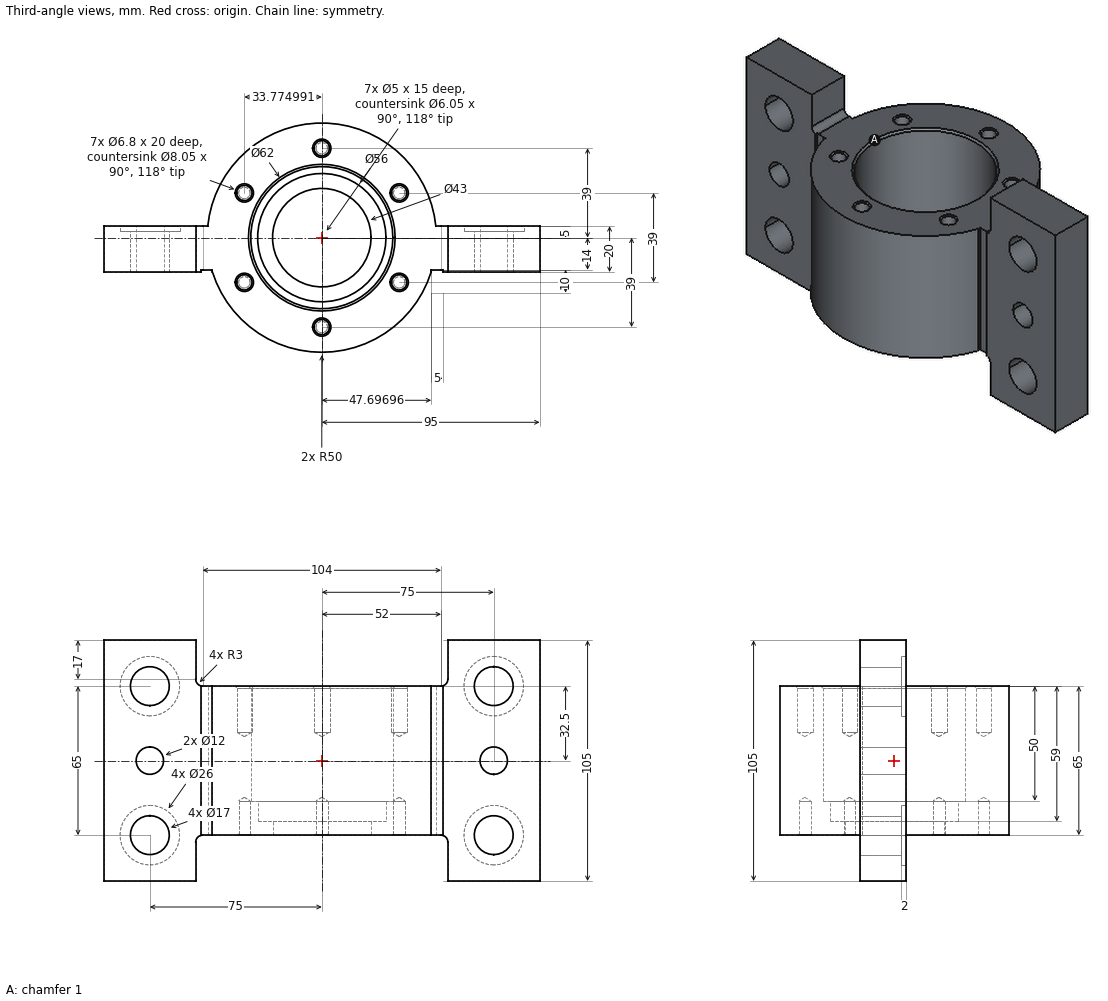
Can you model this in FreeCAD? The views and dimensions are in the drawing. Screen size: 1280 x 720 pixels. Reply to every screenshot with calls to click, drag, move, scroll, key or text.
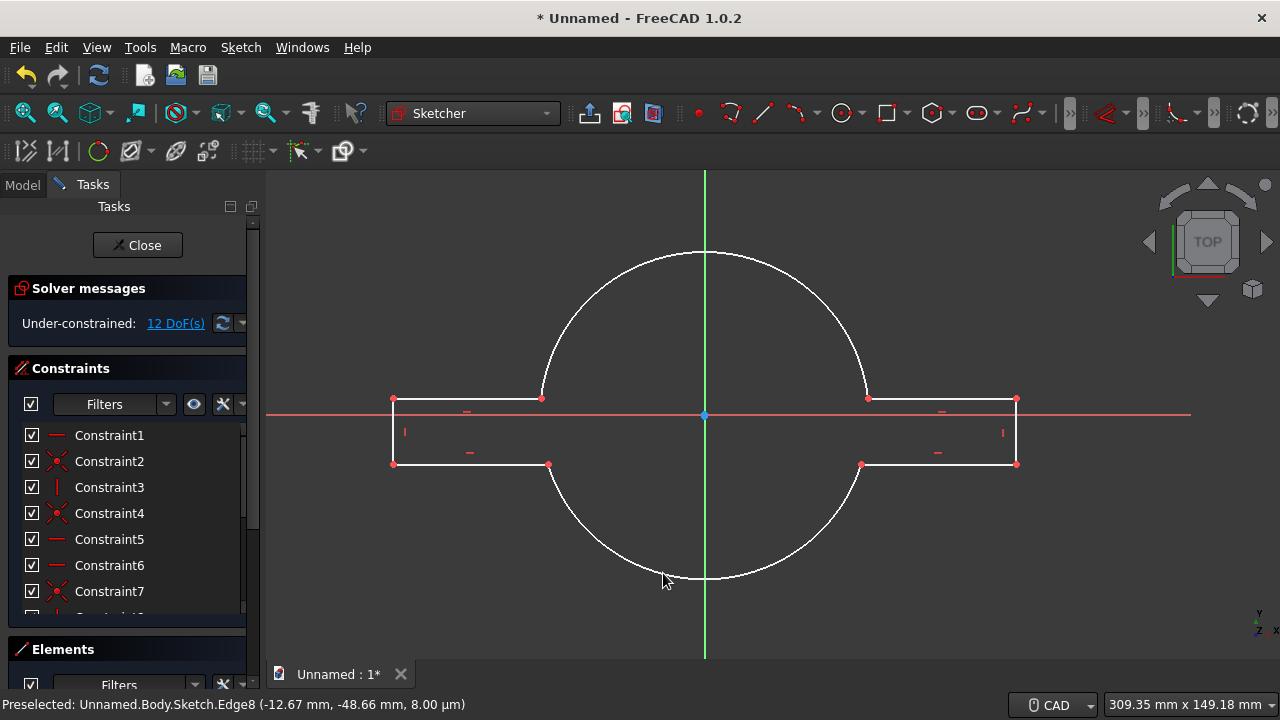
click(795, 279)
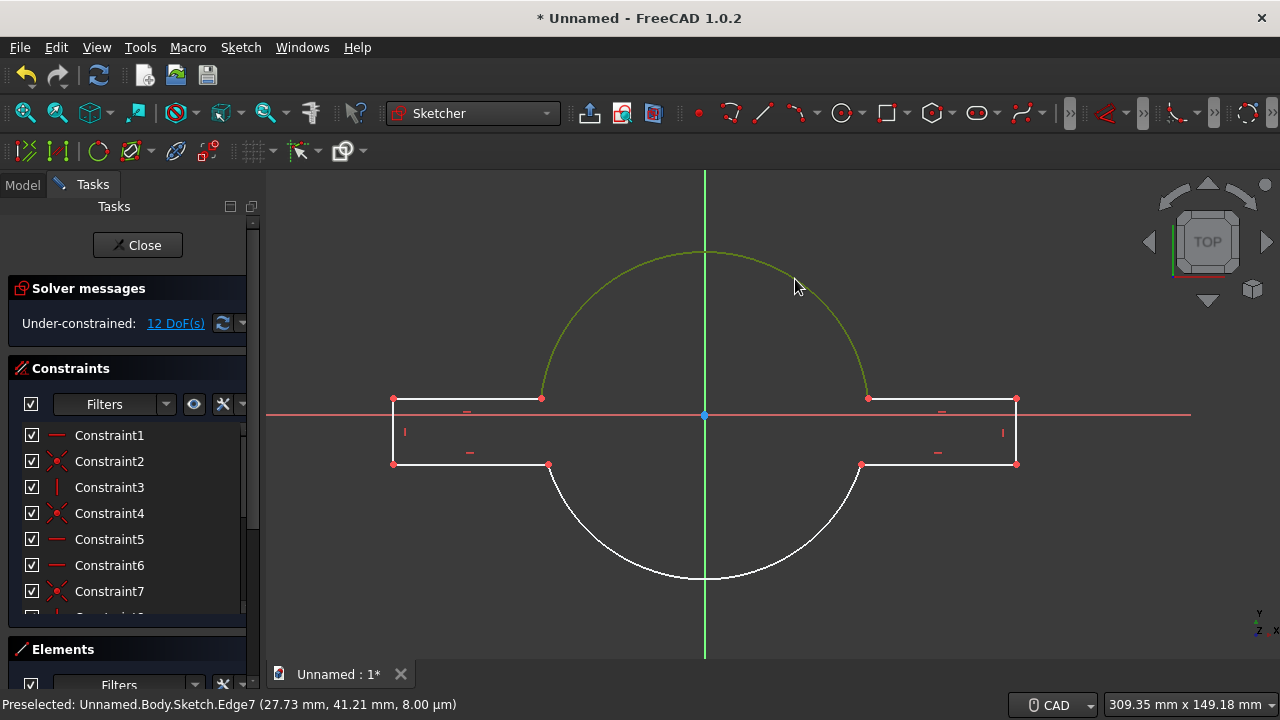
click(625, 559)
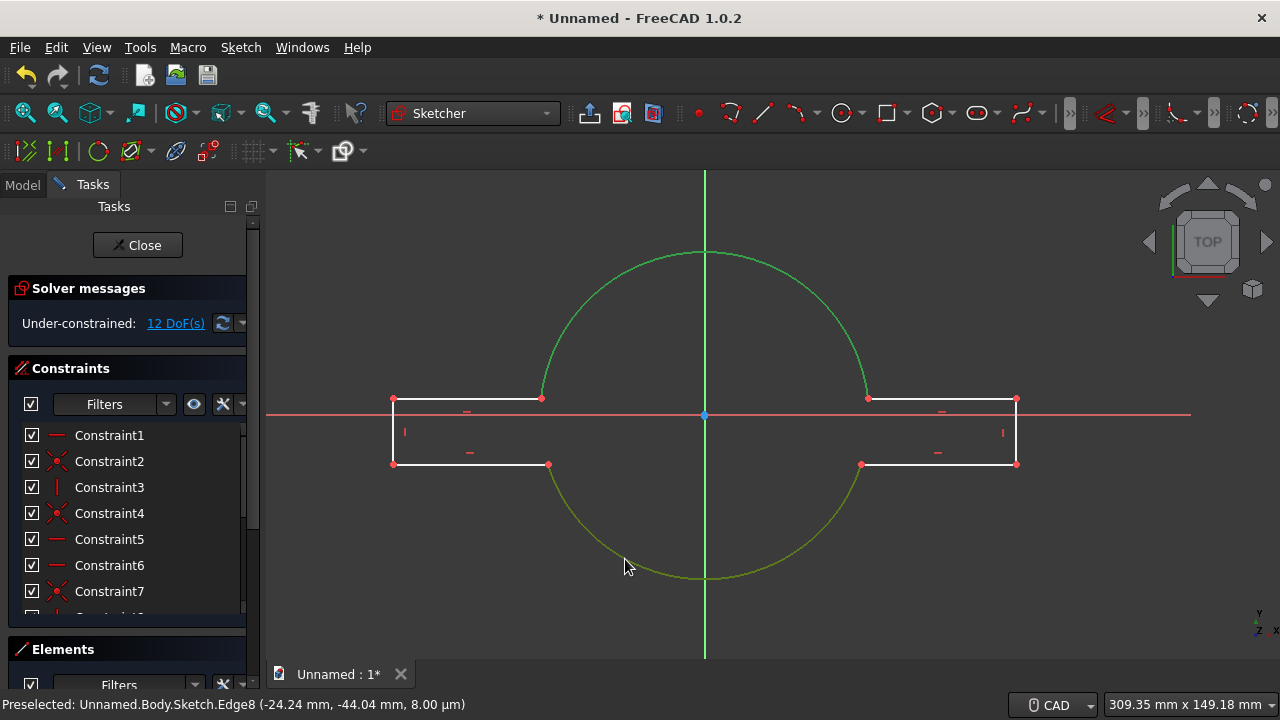
key(c)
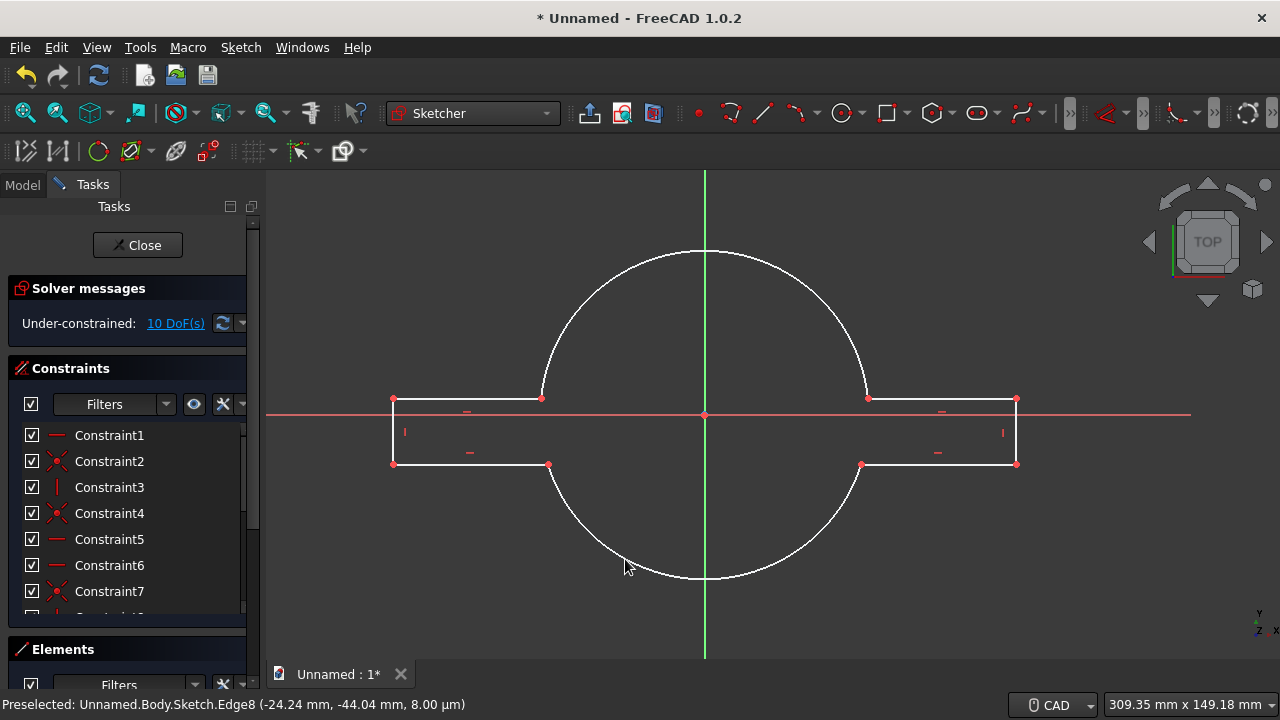
drag(695, 404, 715, 425)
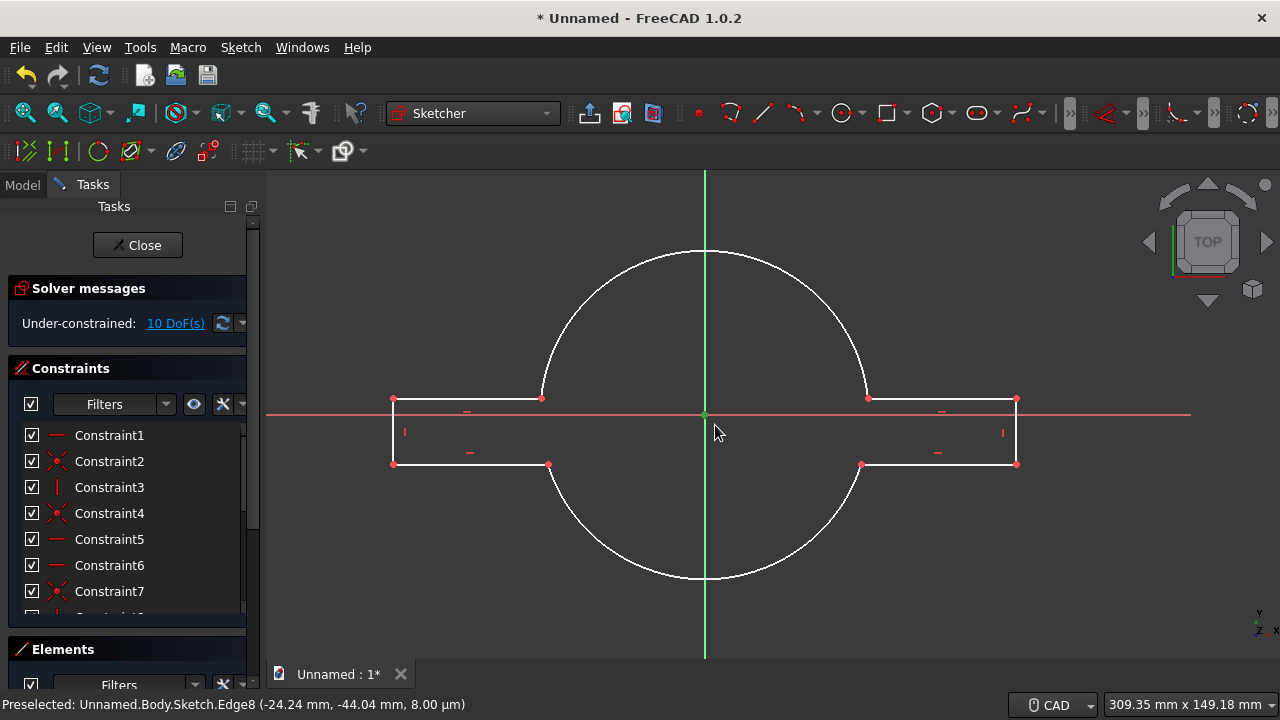
key(c)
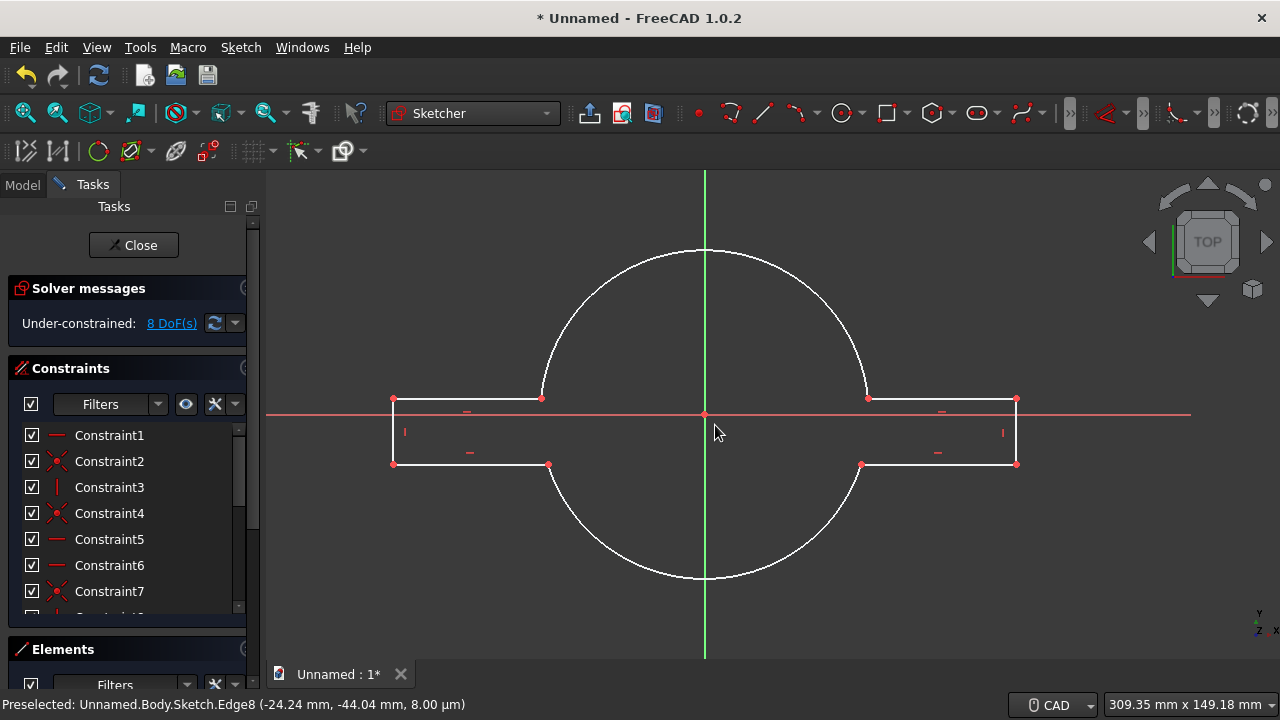
click(796, 278)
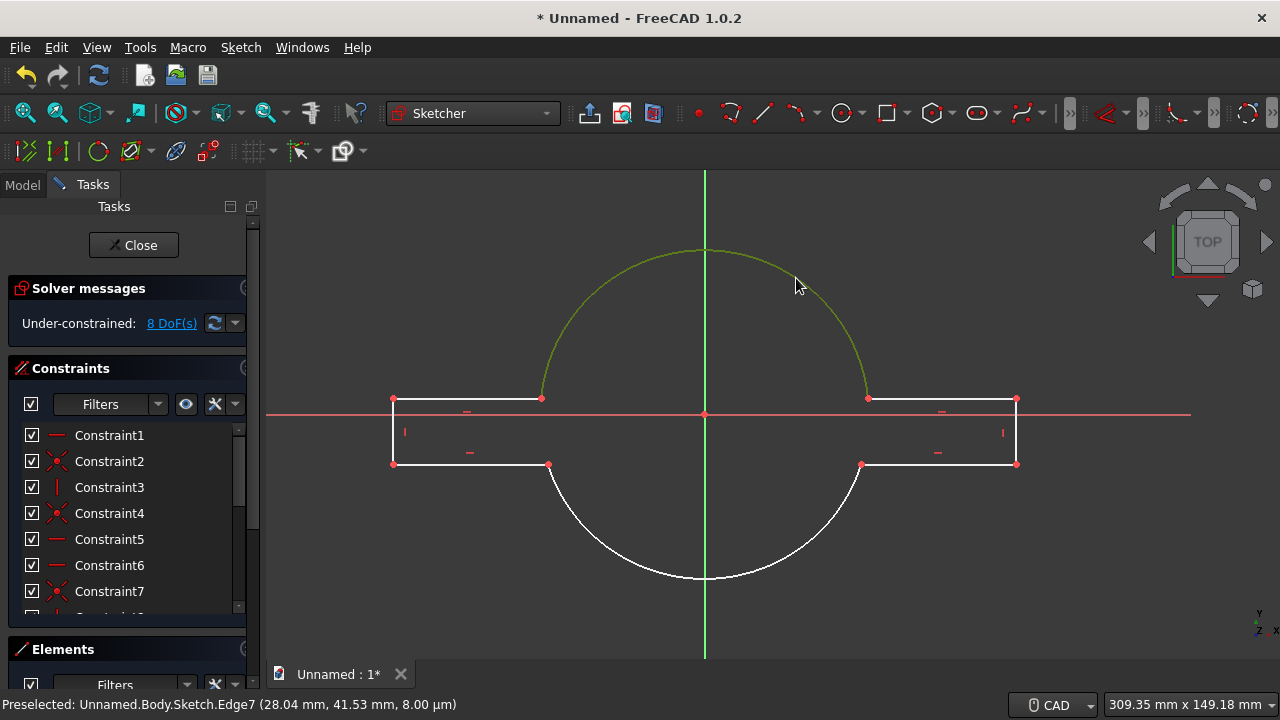
click(625, 559)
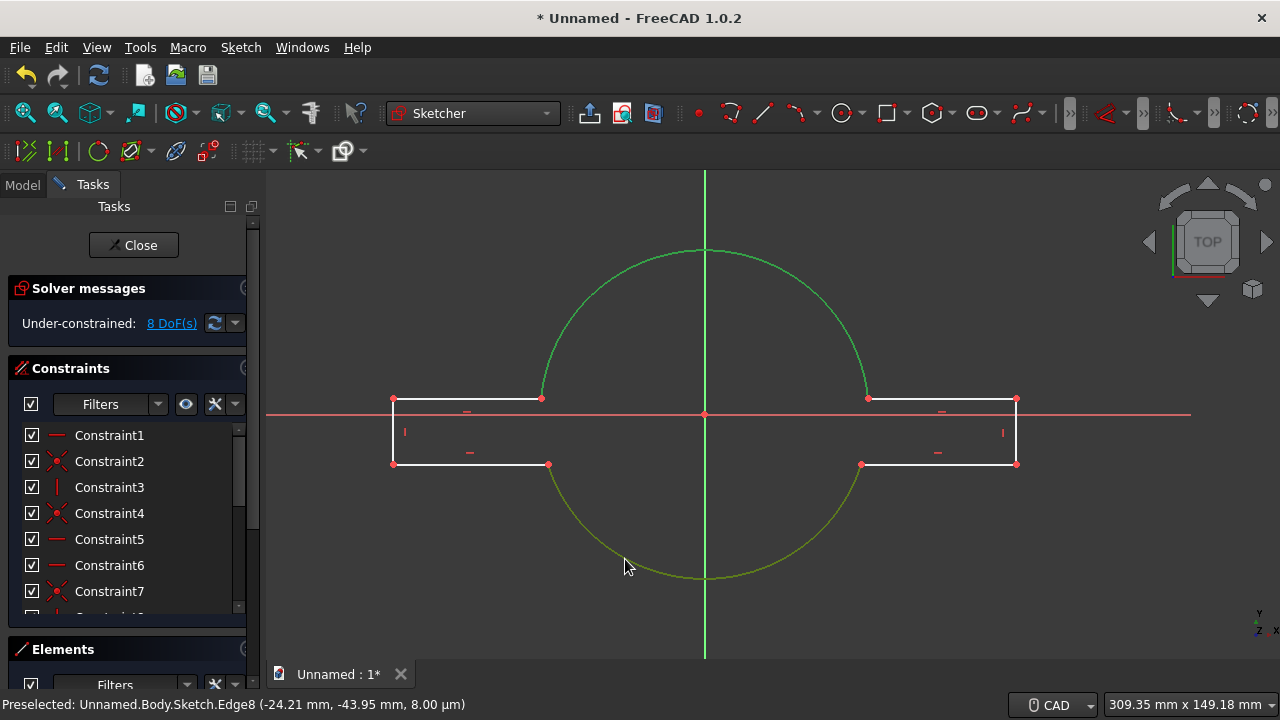
key(e)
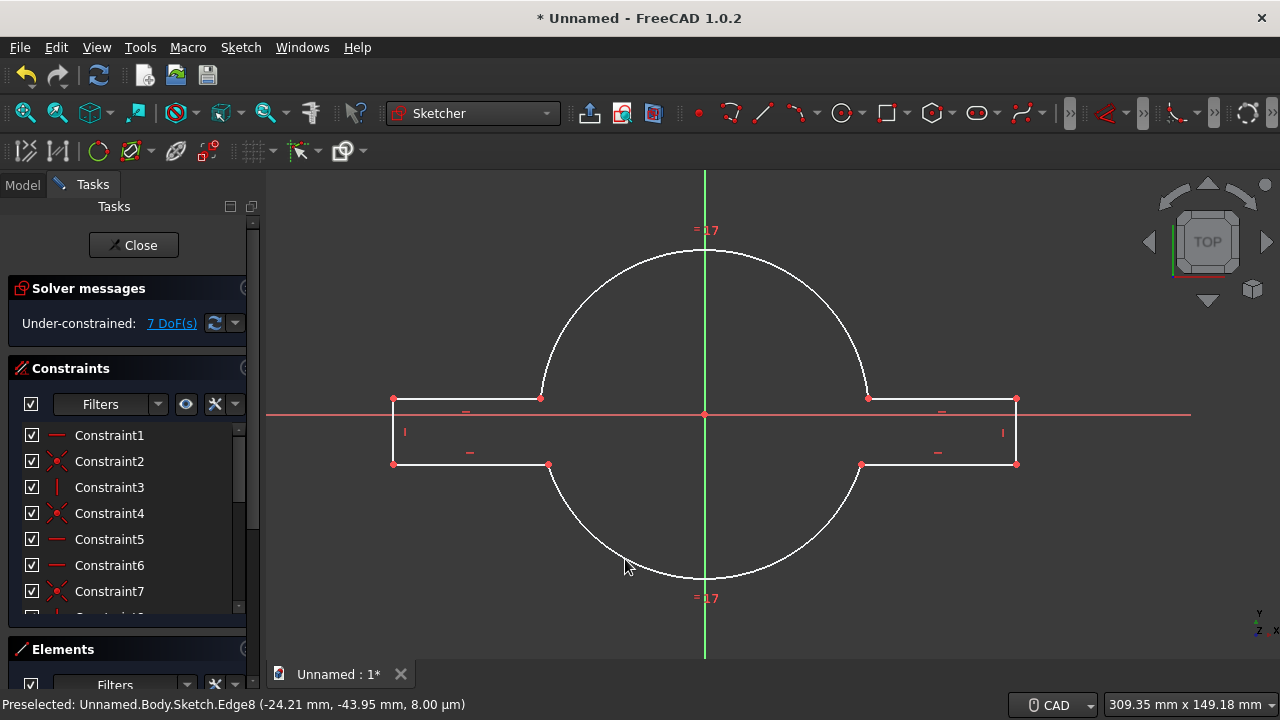
click(1016, 399)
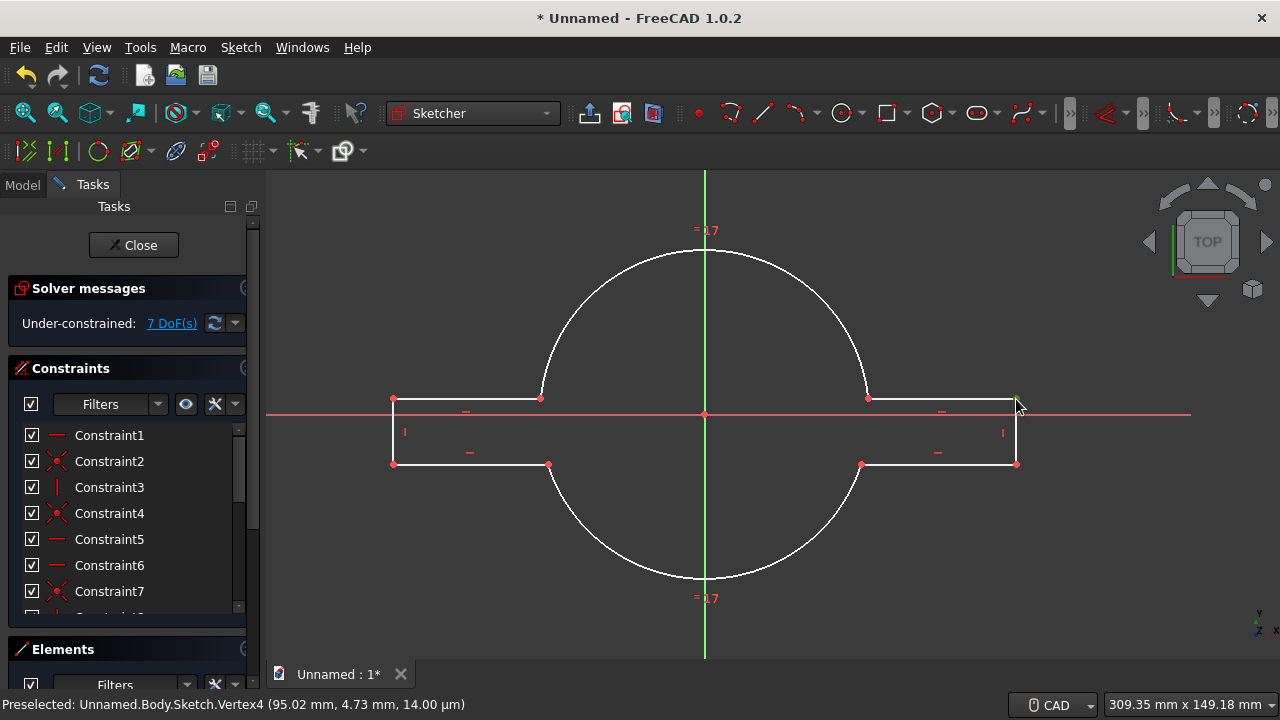
click(393, 399)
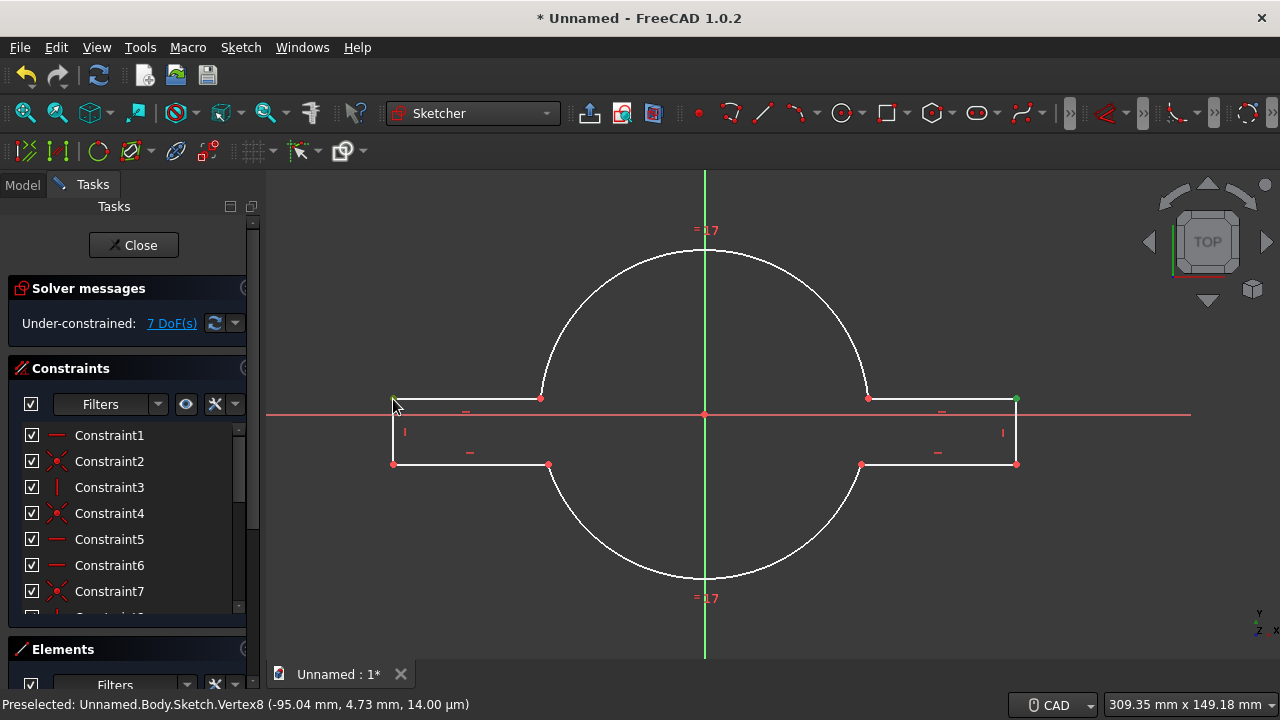
click(705, 538)